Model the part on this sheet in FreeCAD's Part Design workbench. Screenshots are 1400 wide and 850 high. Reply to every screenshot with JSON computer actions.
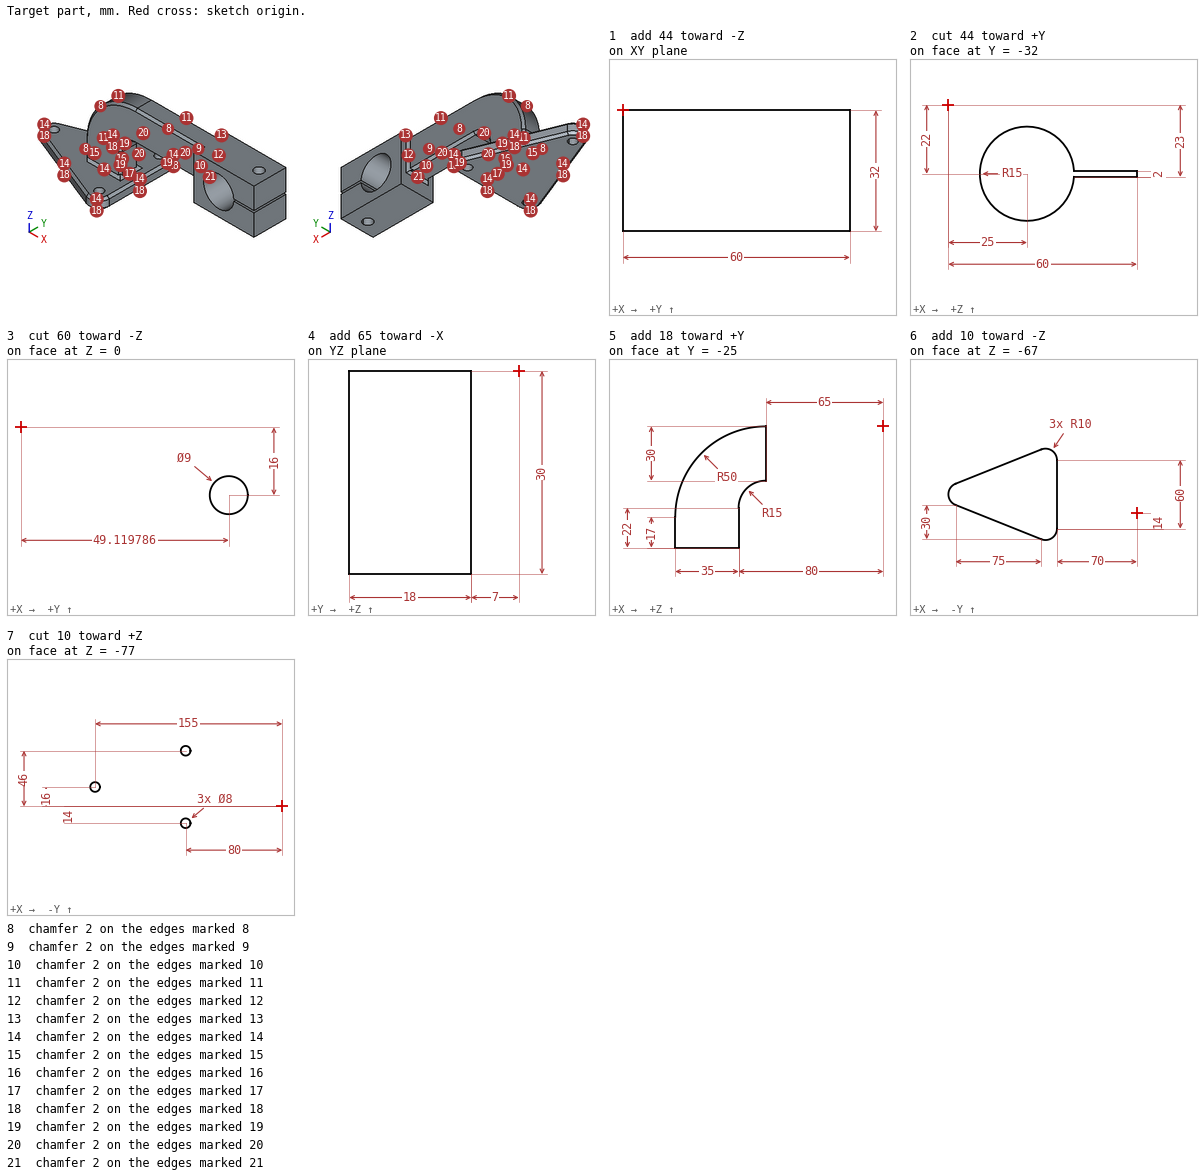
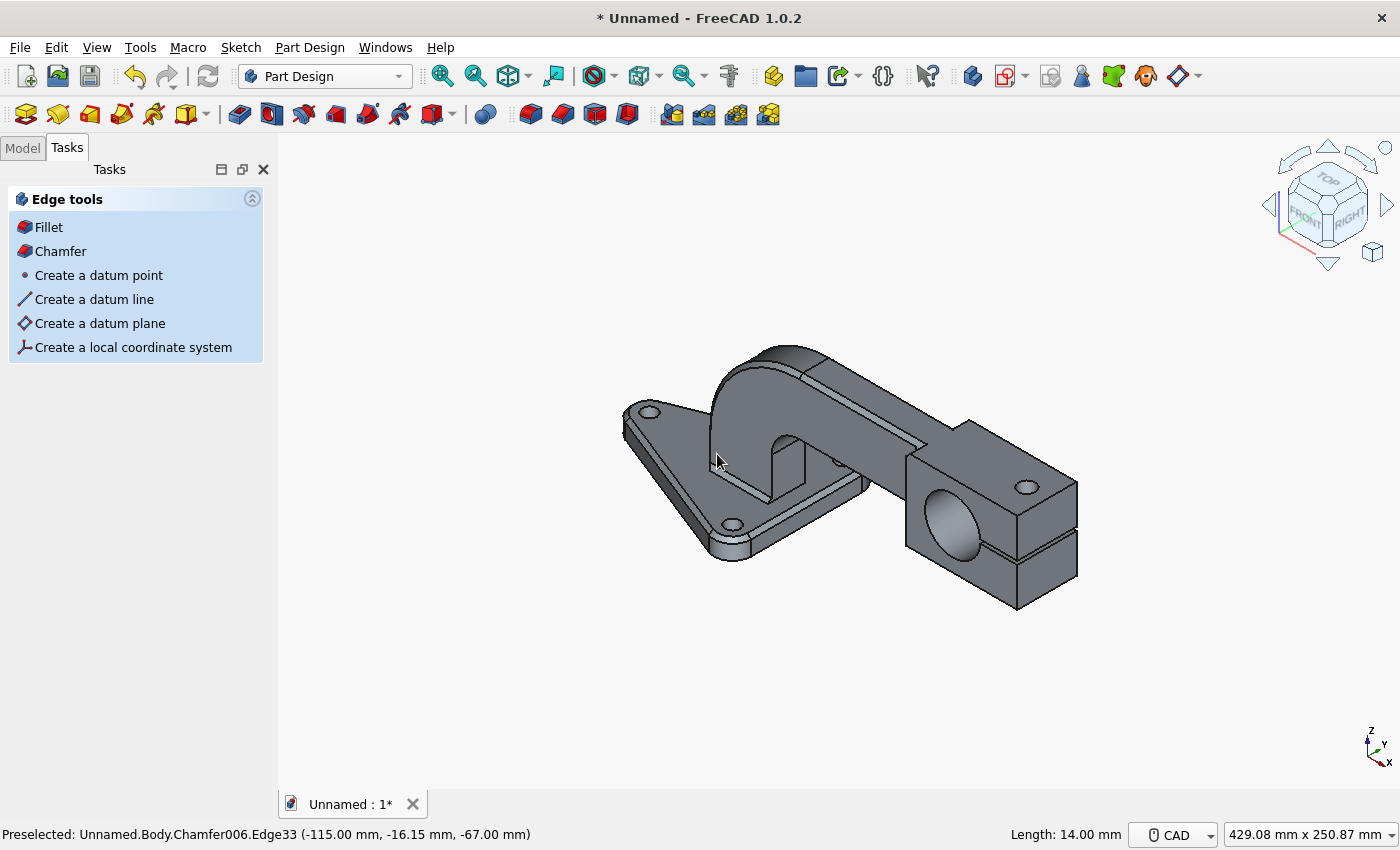
{"action": "left_click", "coordinate": [564, 114]}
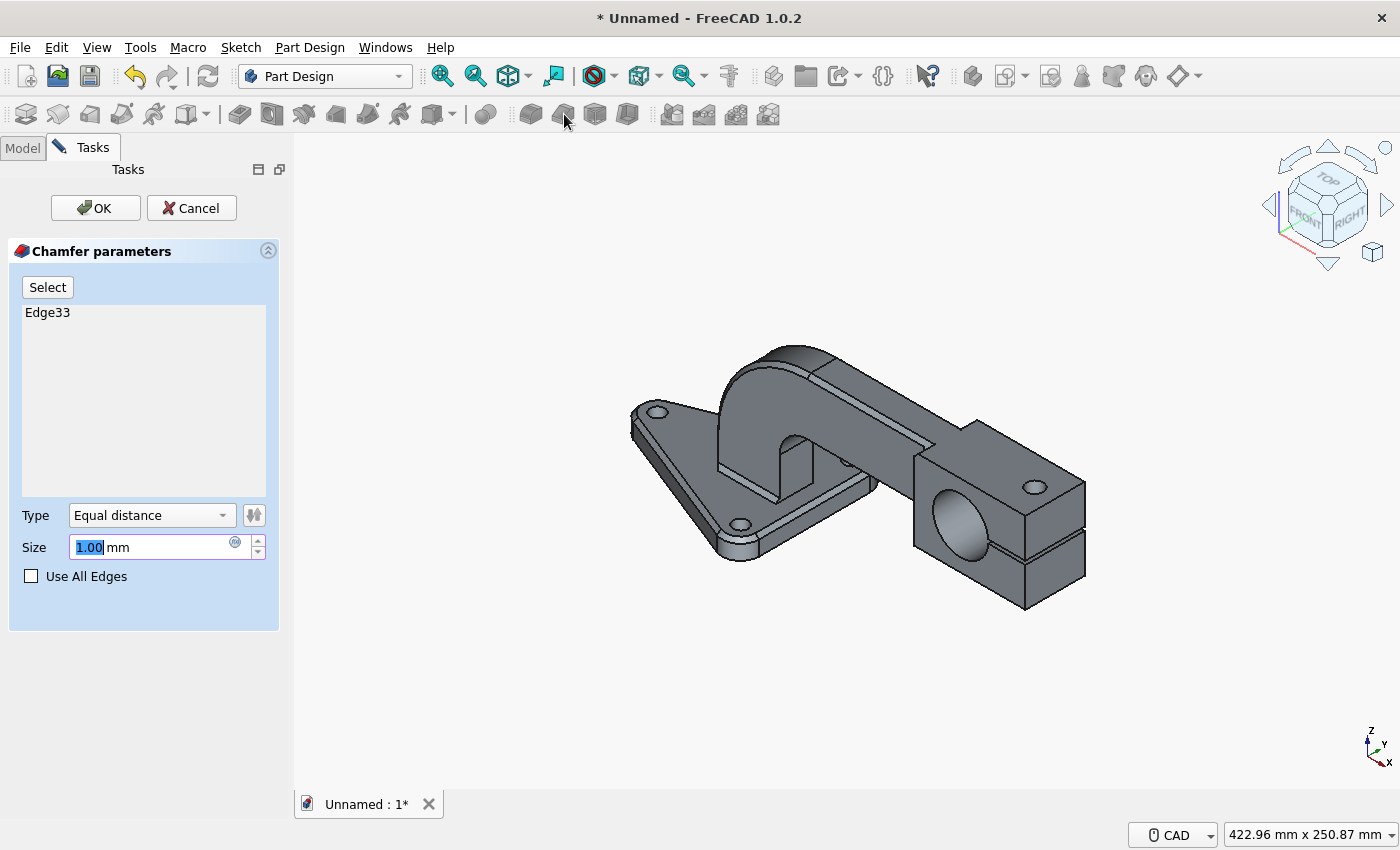
{"action": "type", "text": "2"}
{"action": "key", "text": "Tab"}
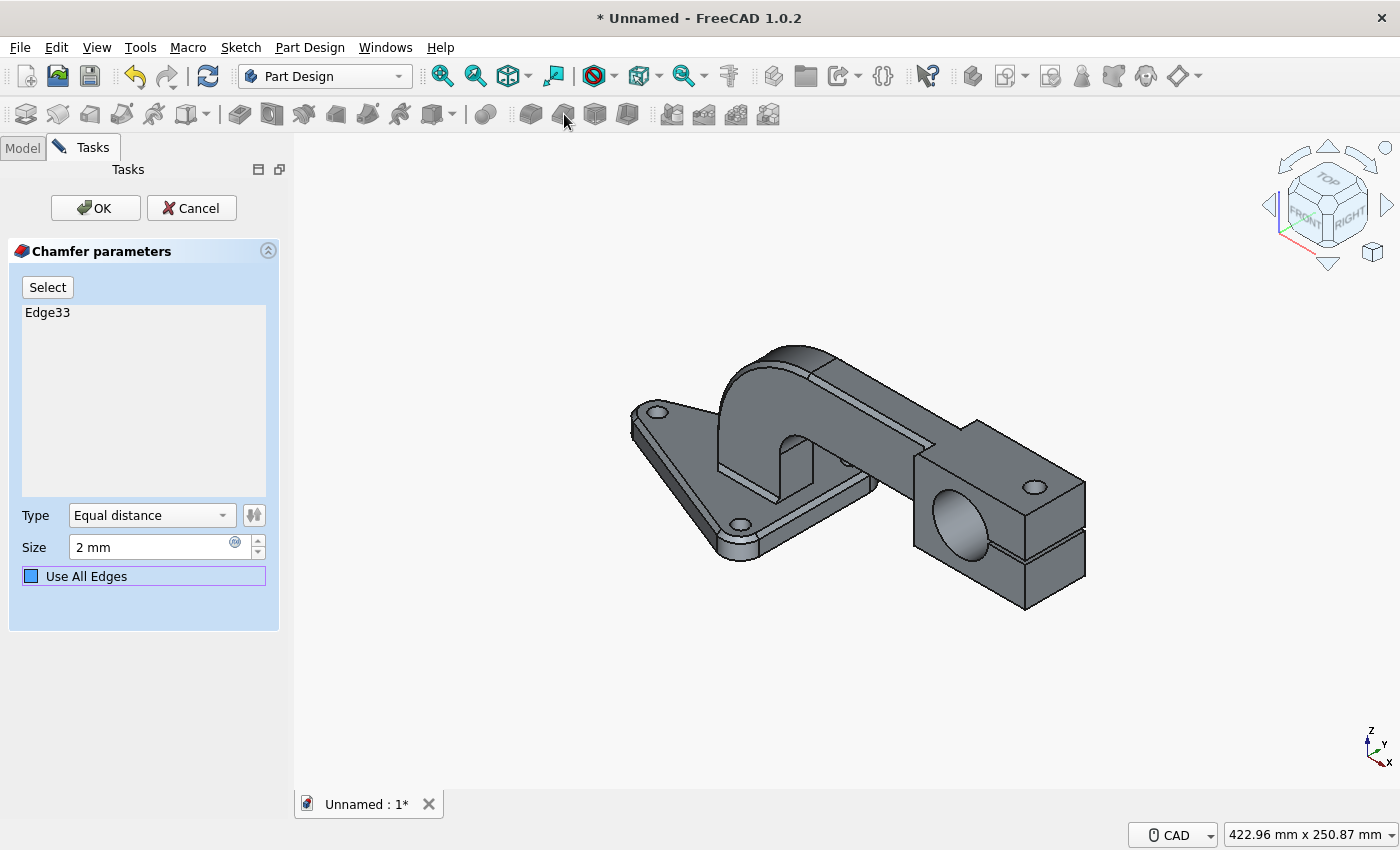
{"action": "left_click", "coordinate": [96, 208]}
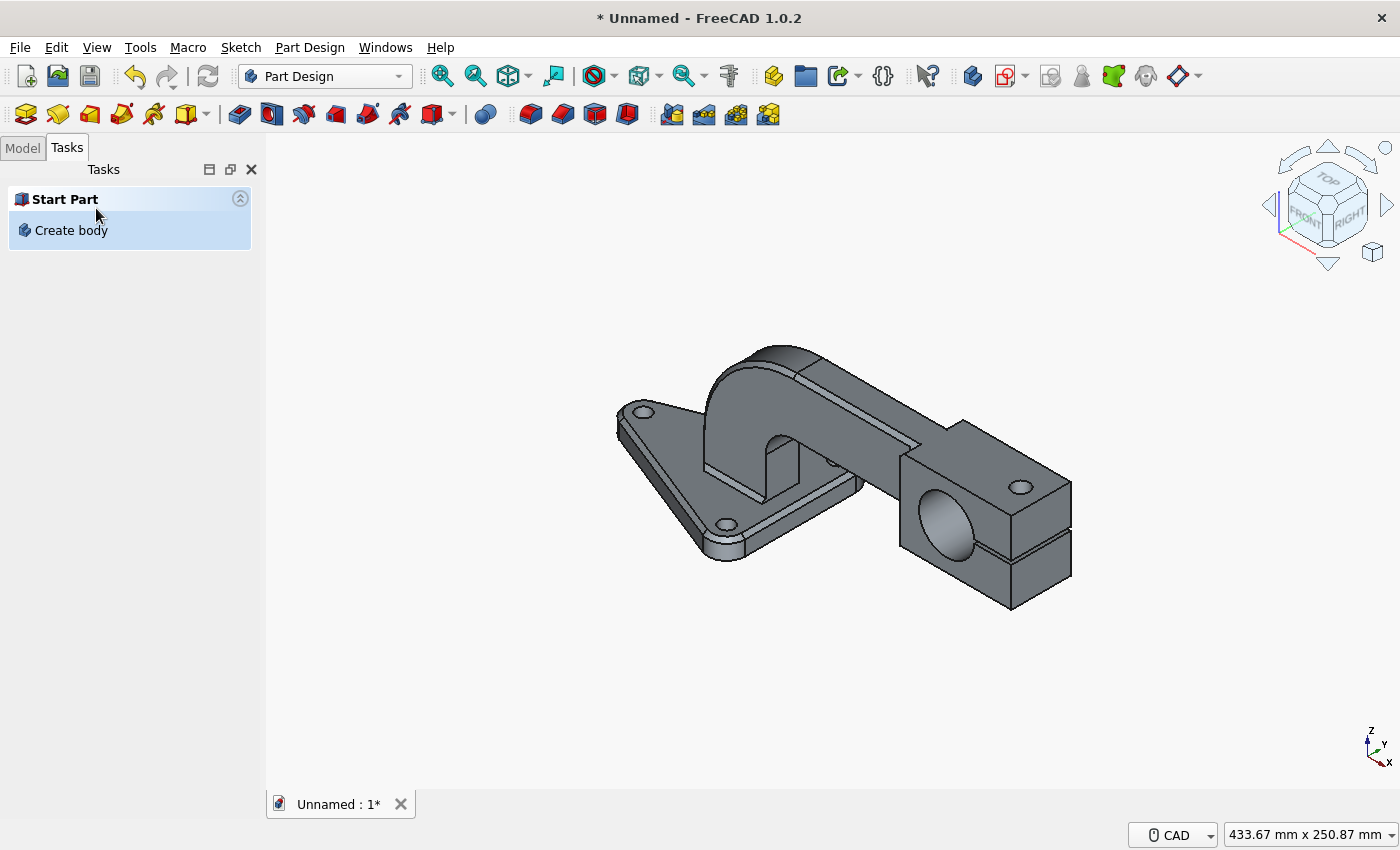
{"action": "key", "text": "2"}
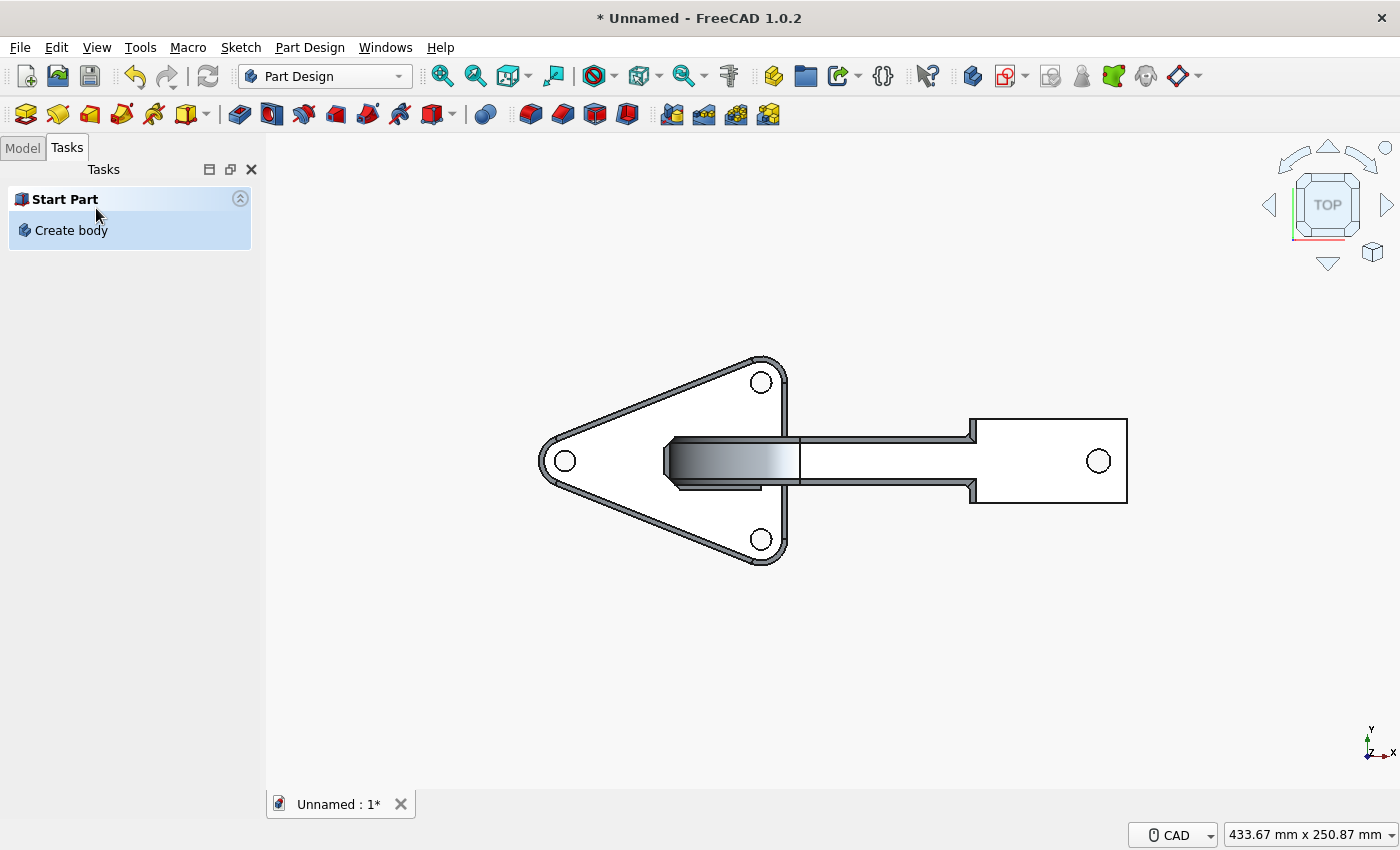
{"action": "key", "text": "0"}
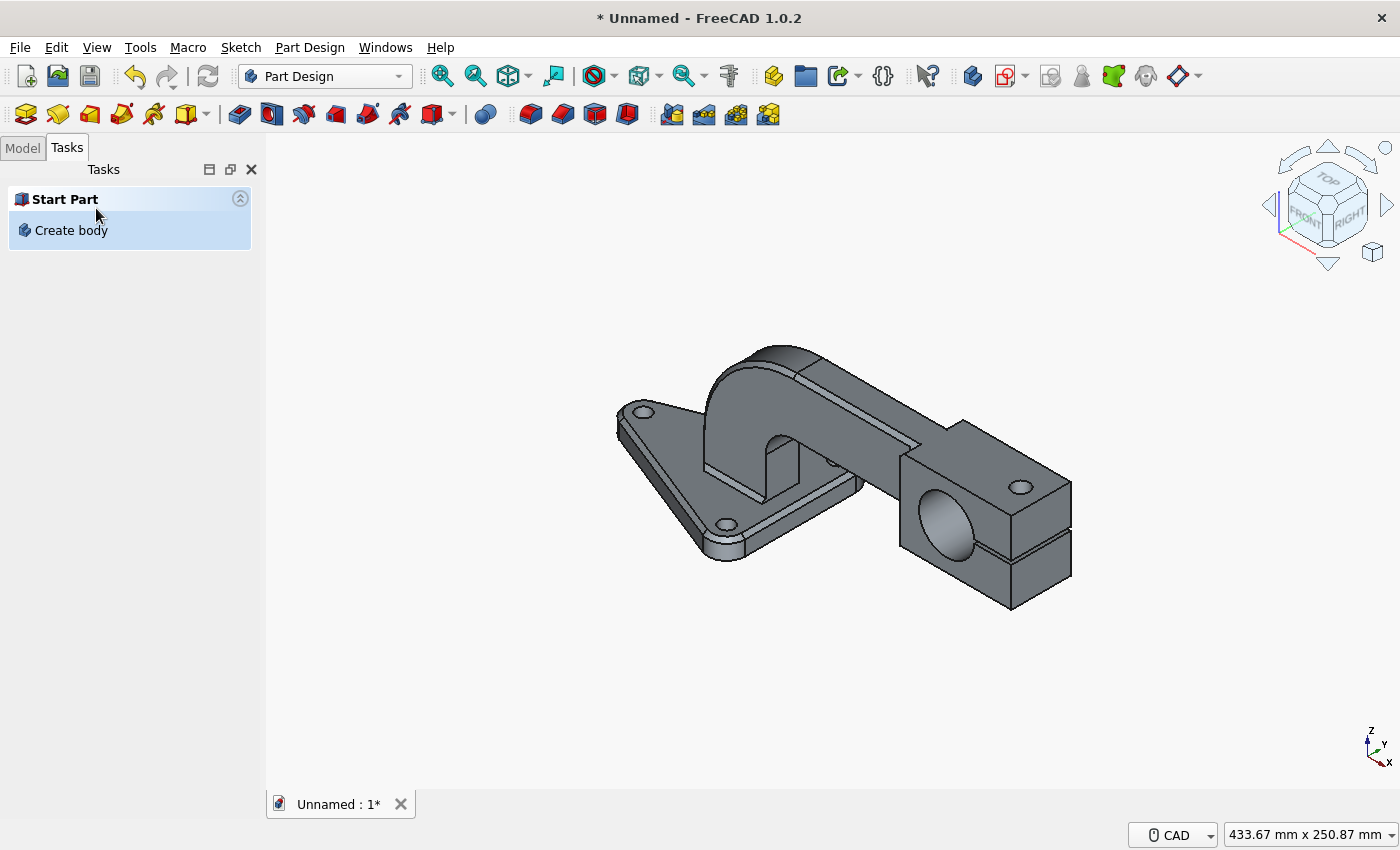
{"action": "key", "text": "1"}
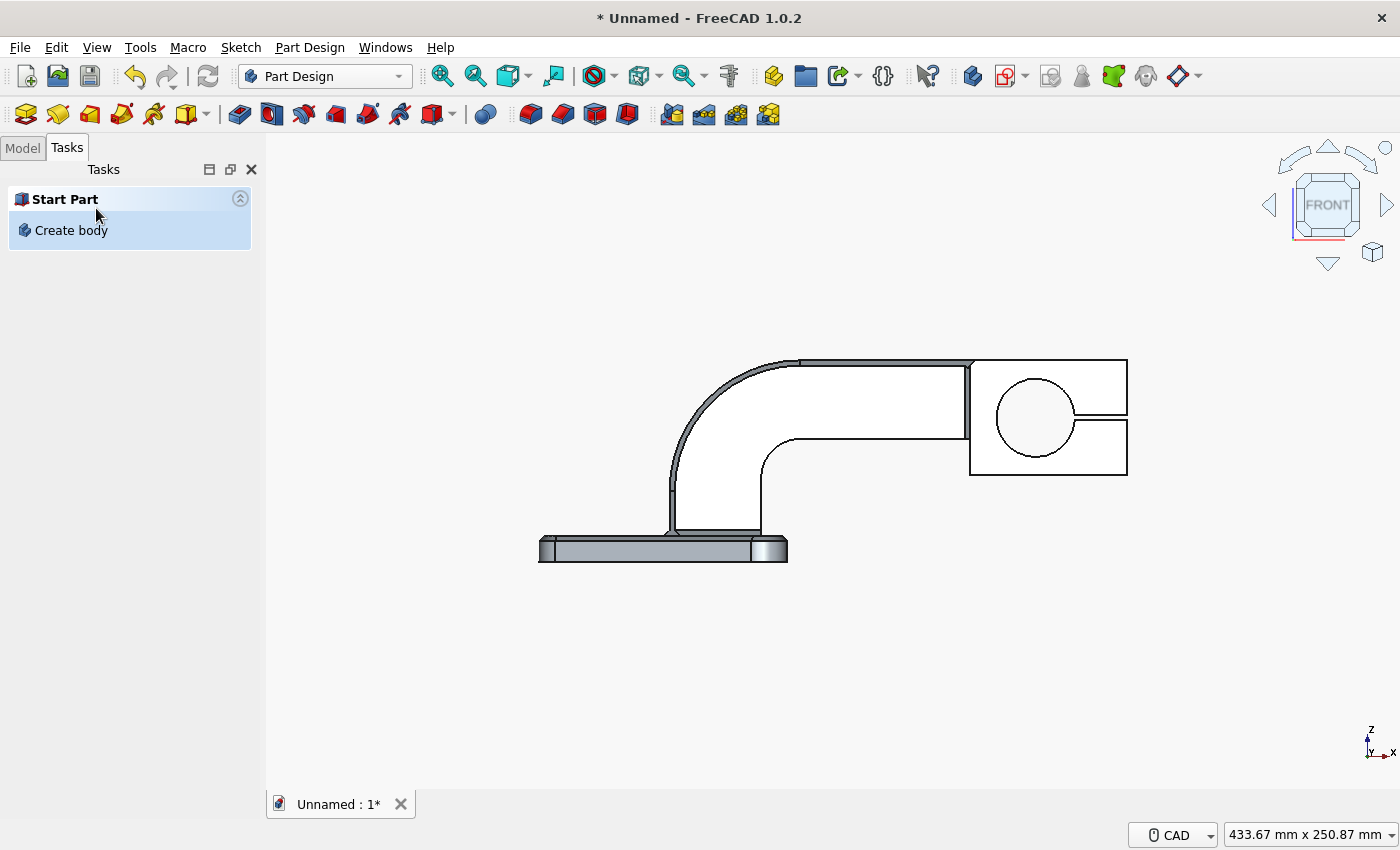
{"action": "key", "text": "3"}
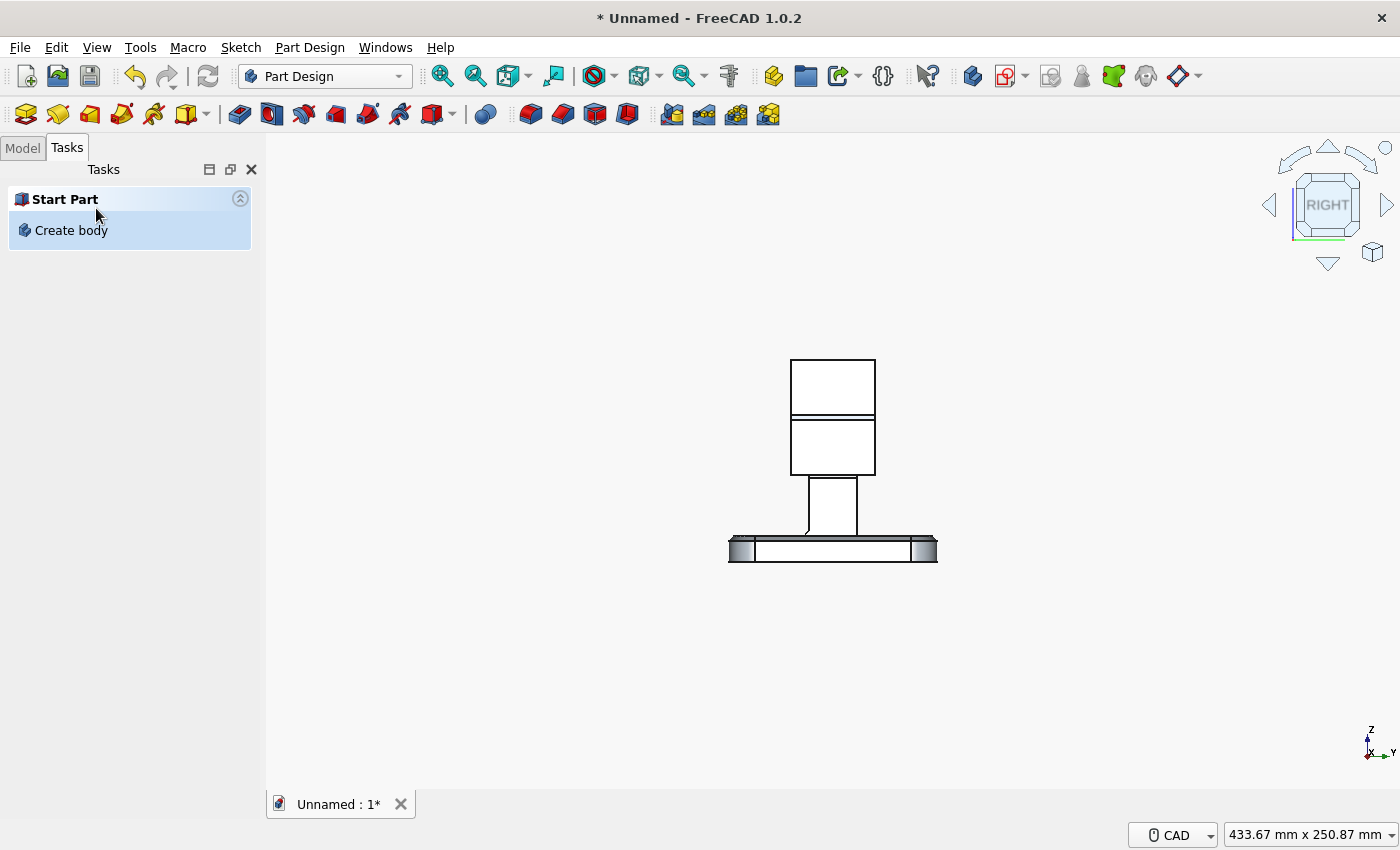
{"action": "key", "text": "v f"}